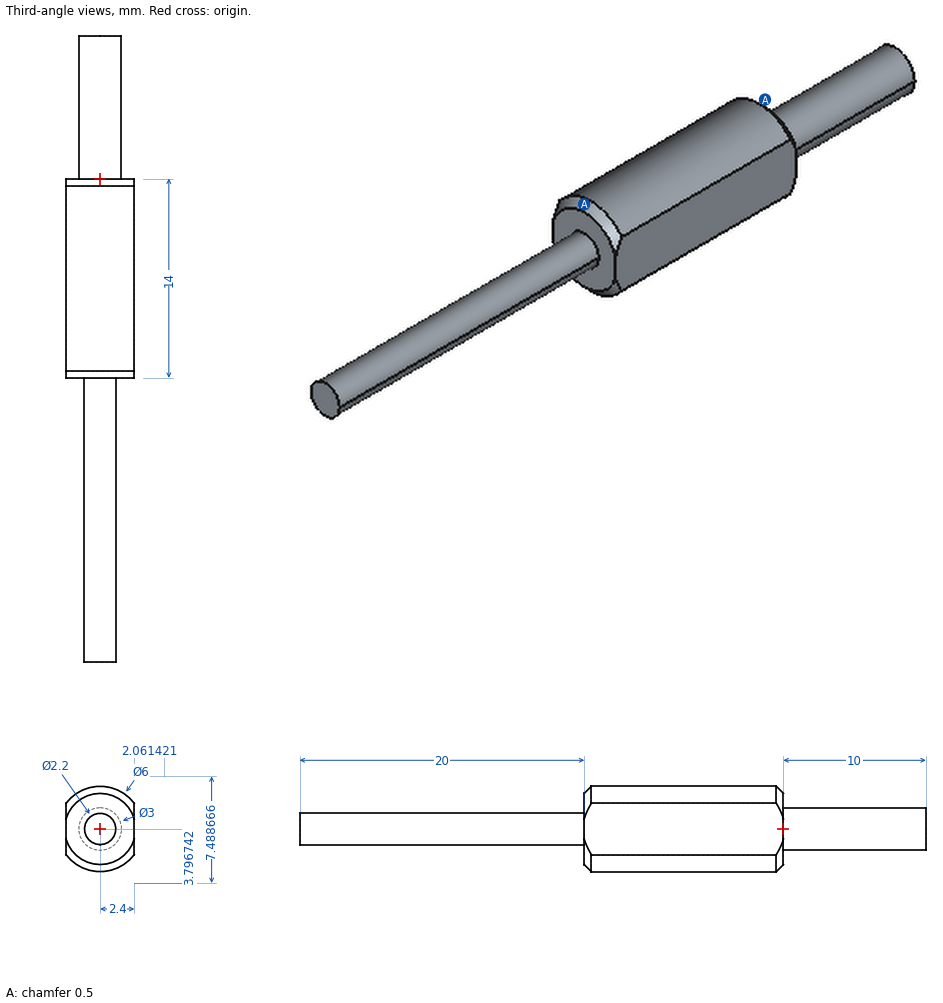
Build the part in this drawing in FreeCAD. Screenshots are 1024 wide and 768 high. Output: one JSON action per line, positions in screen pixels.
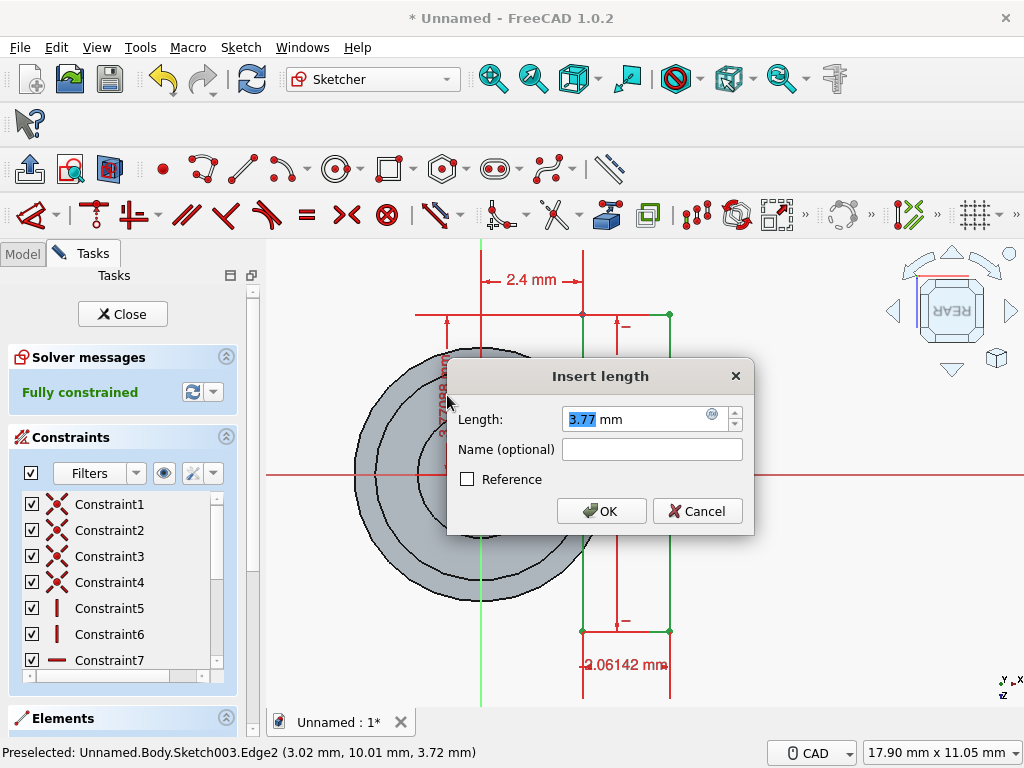
{"action": "type", "text": "3.796742"}
{"action": "key", "text": "Return"}
{"action": "key", "text": "Escape"}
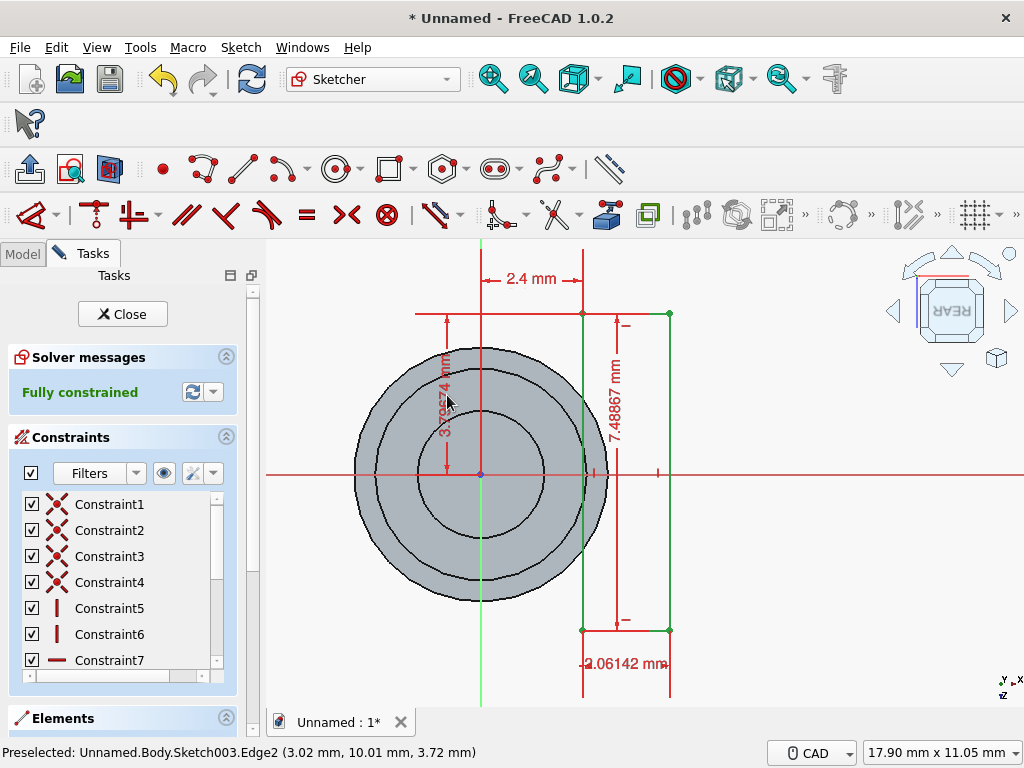
{"action": "left_click", "coordinate": [123, 314]}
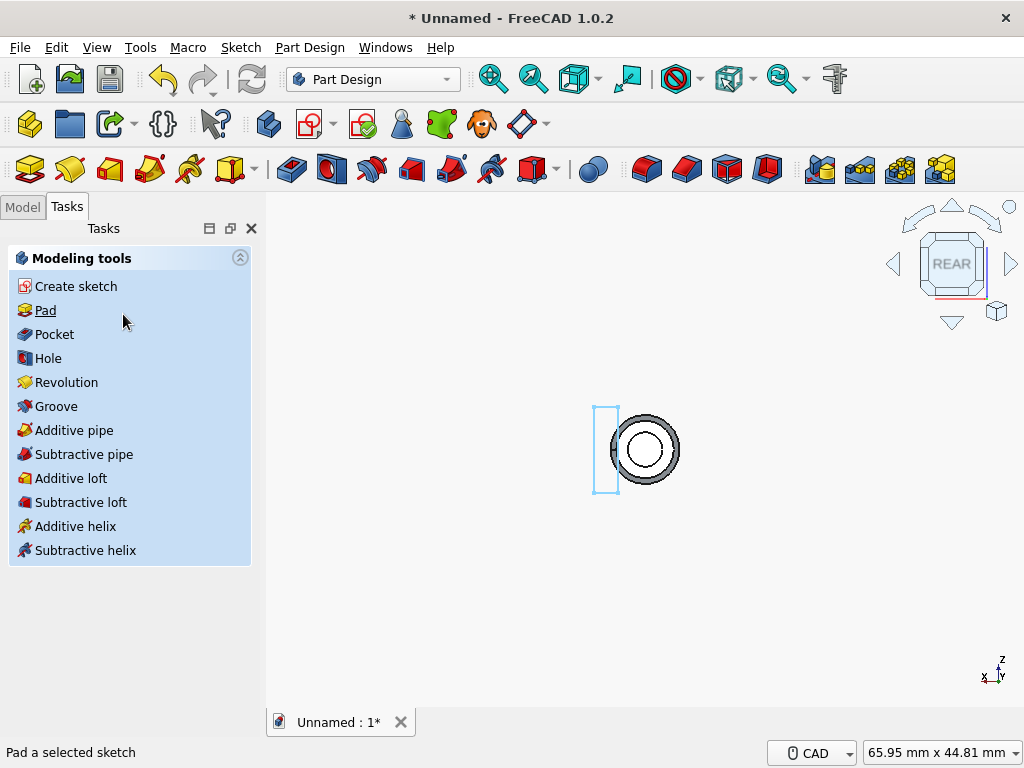
{"action": "left_click", "coordinate": [292, 170]}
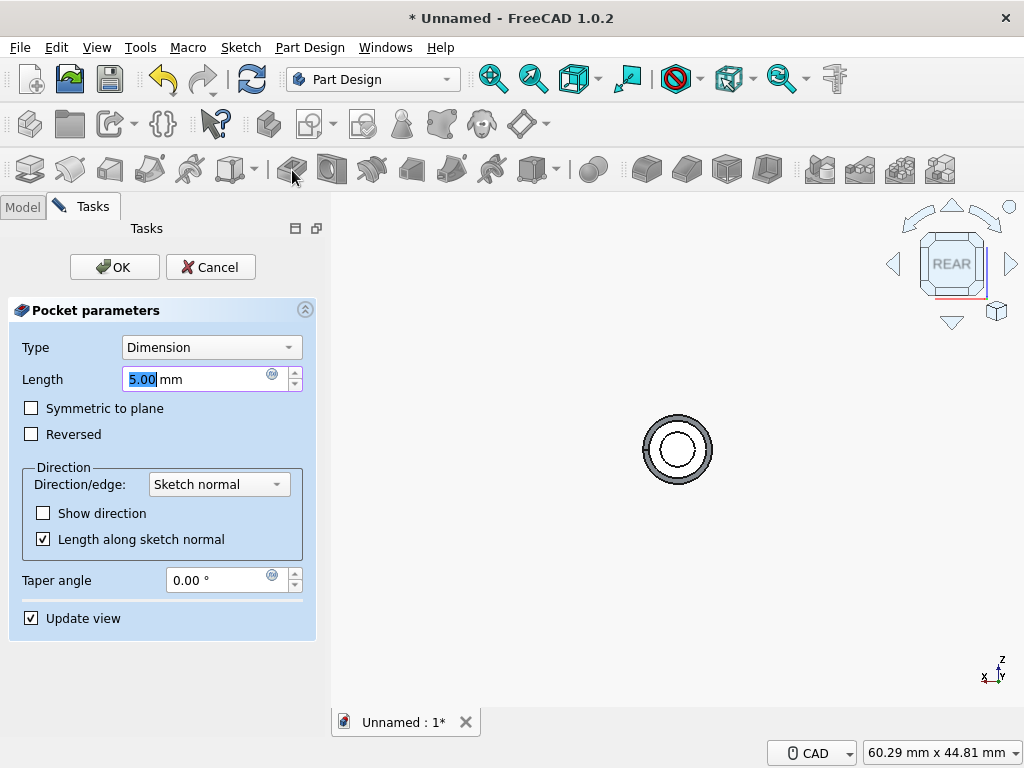
{"action": "left_click", "coordinate": [212, 348]}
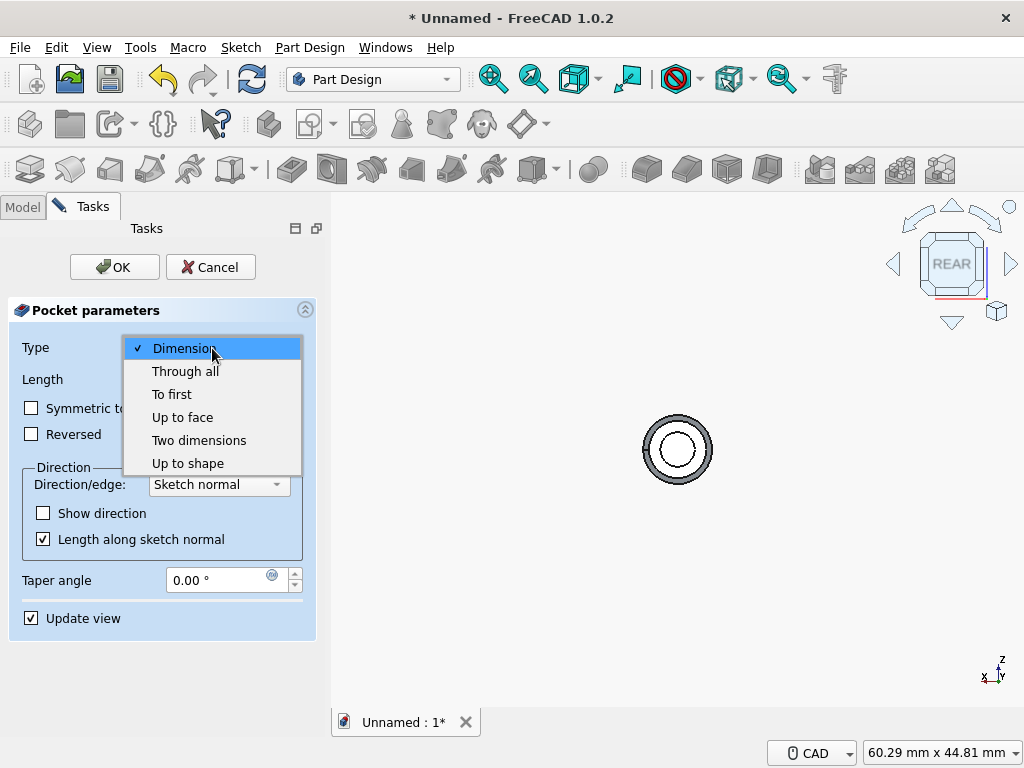
{"action": "left_click", "coordinate": [212, 372]}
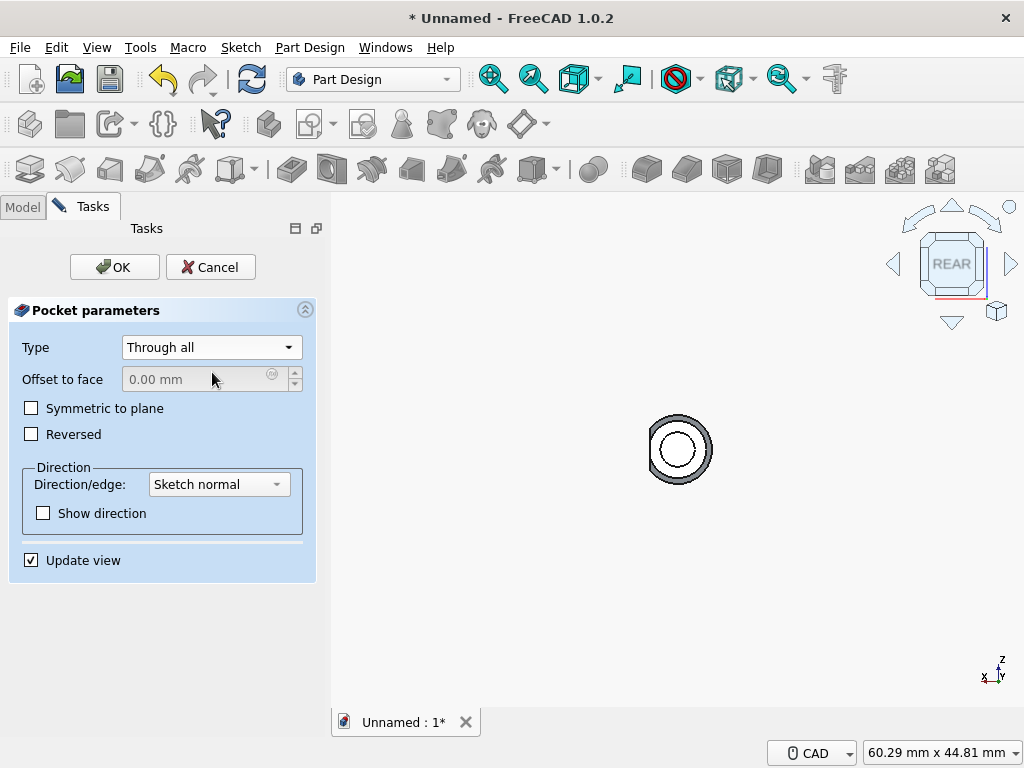
{"action": "left_click", "coordinate": [115, 267]}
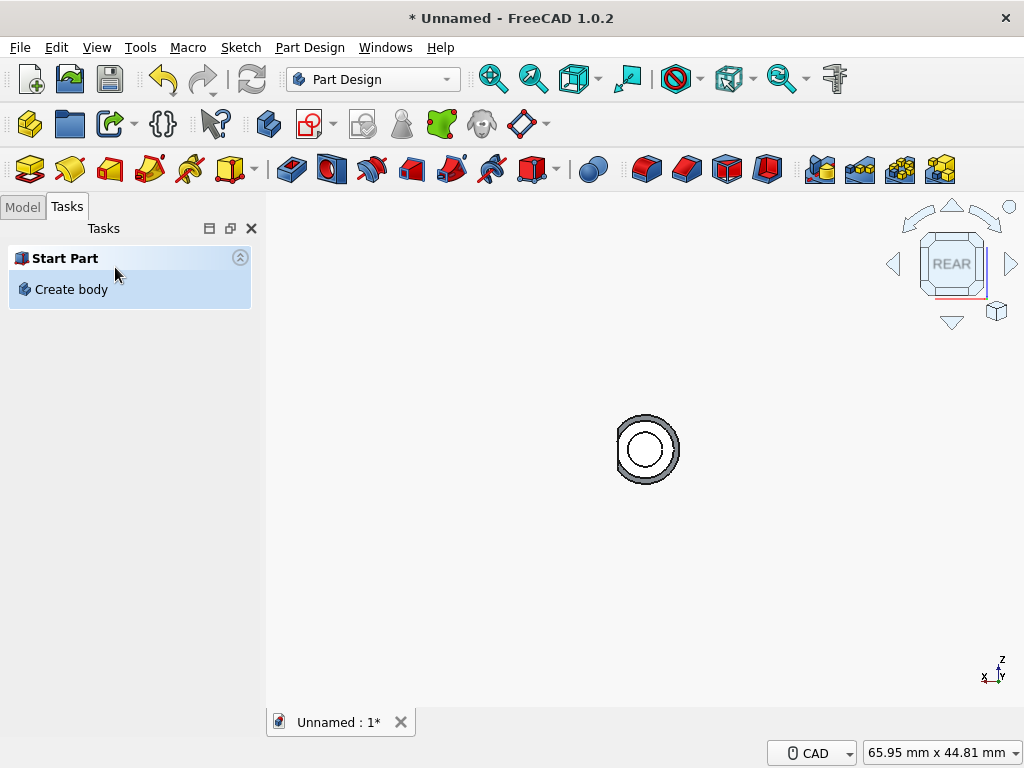
{"action": "left_click", "coordinate": [494, 80]}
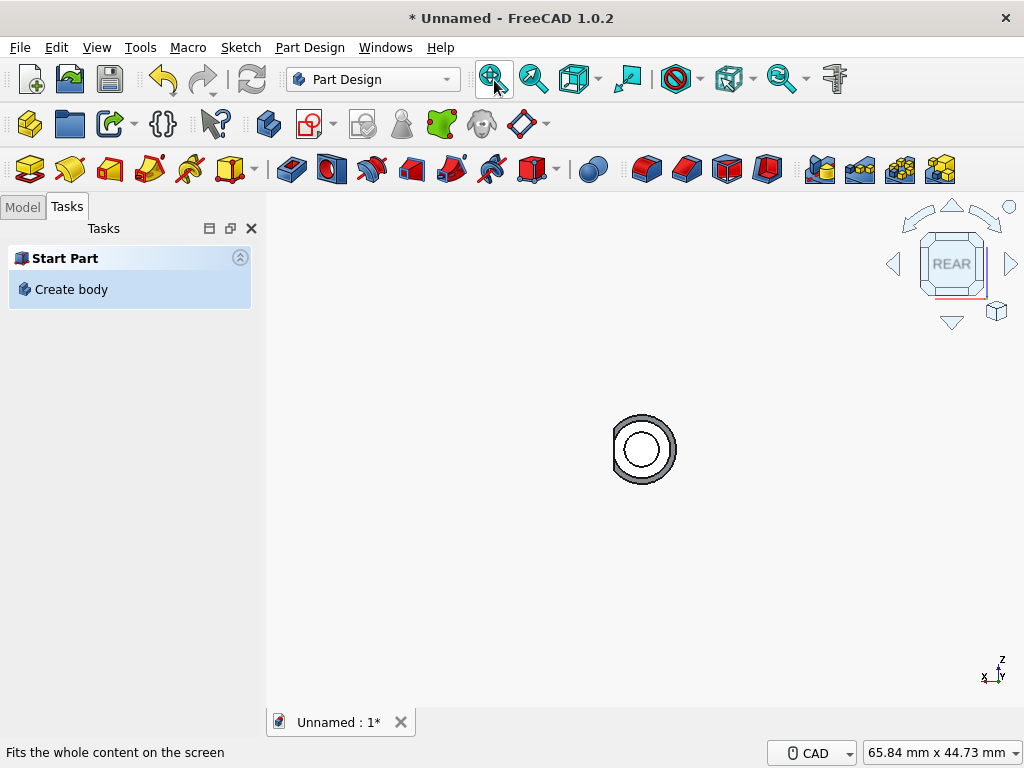
{"action": "left_click", "coordinate": [23, 206]}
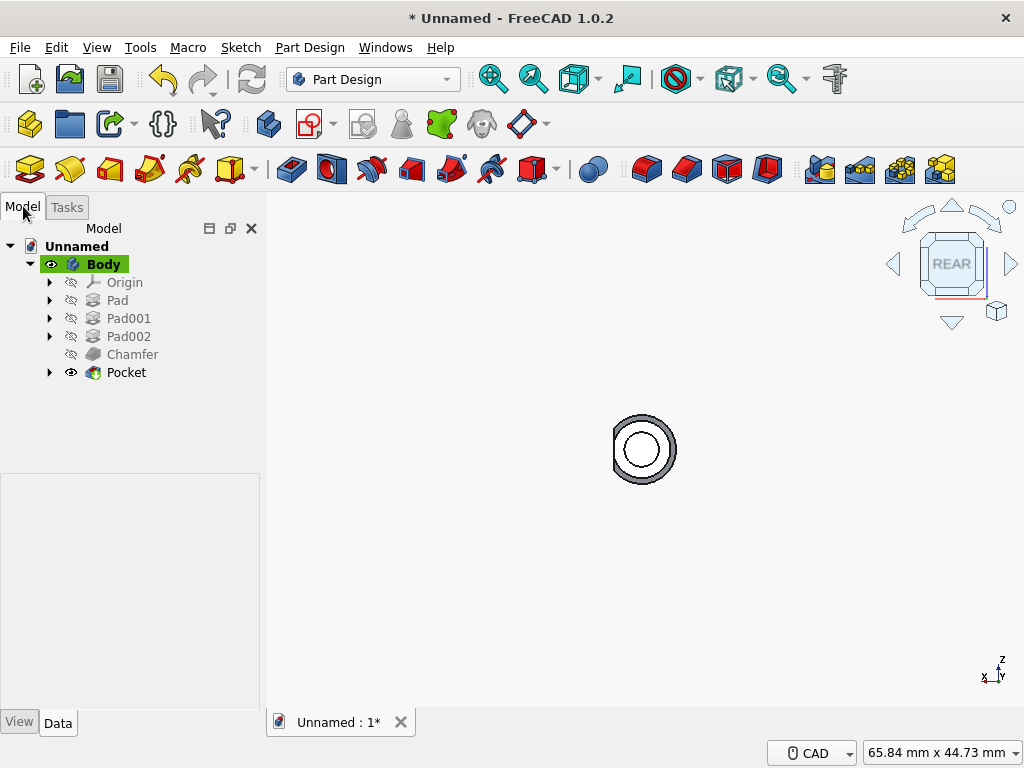
{"action": "left_click", "coordinate": [116, 372]}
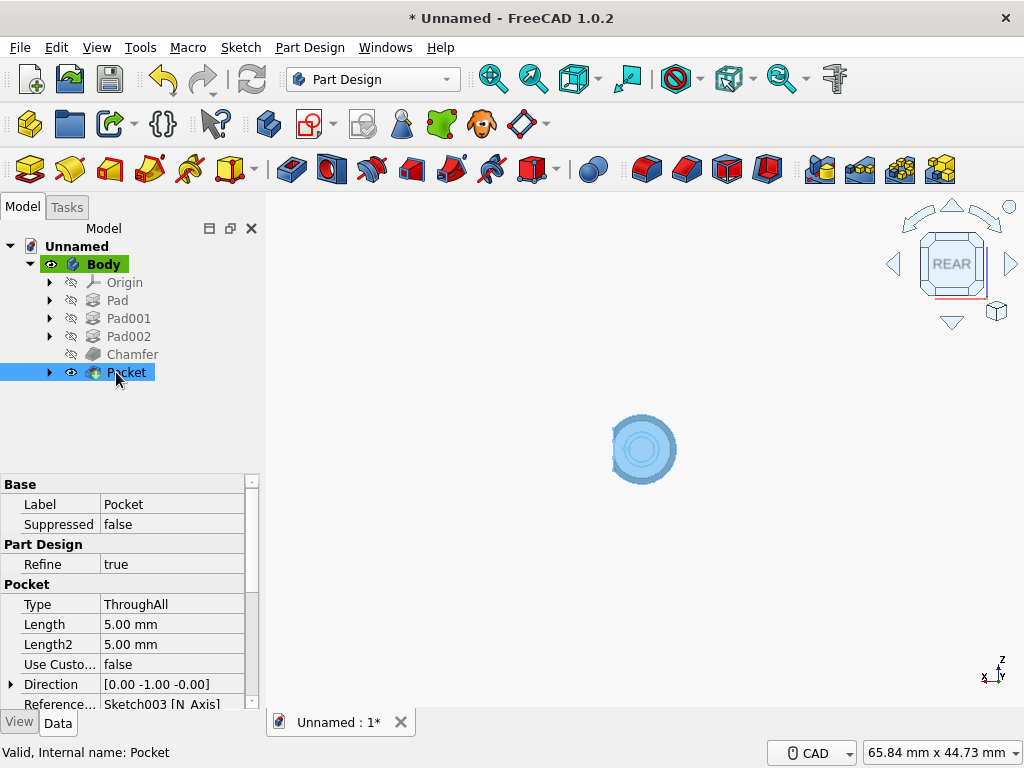
{"action": "left_click", "coordinate": [820, 170]}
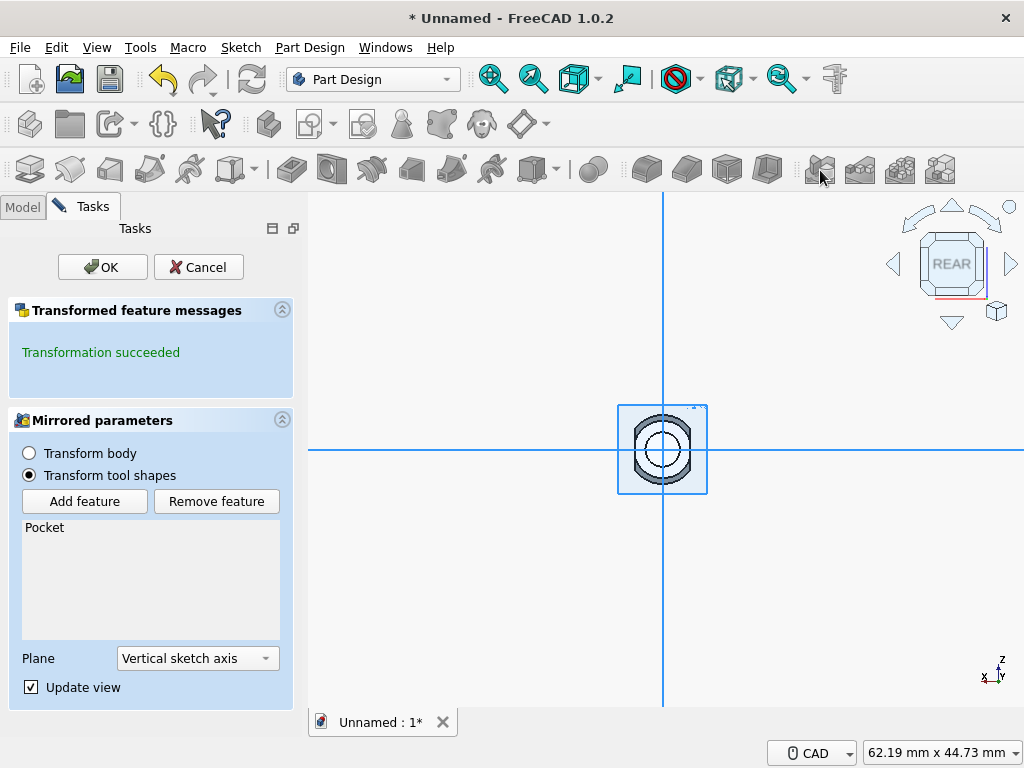
{"action": "left_click", "coordinate": [198, 658]}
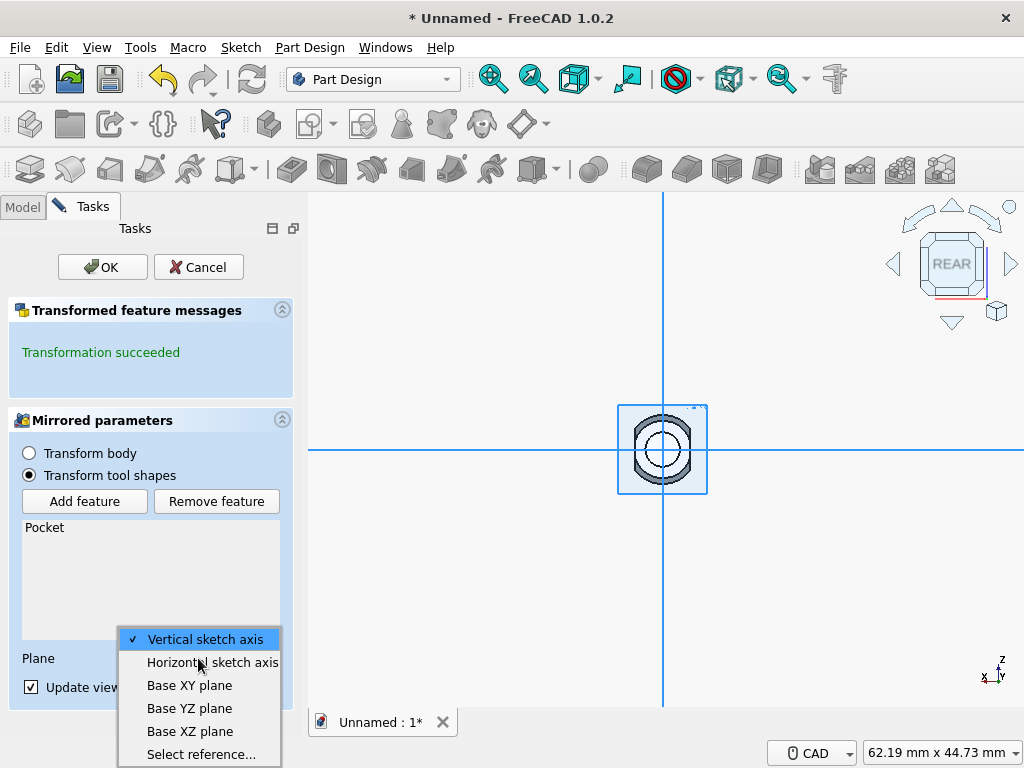
{"action": "left_click", "coordinate": [198, 708]}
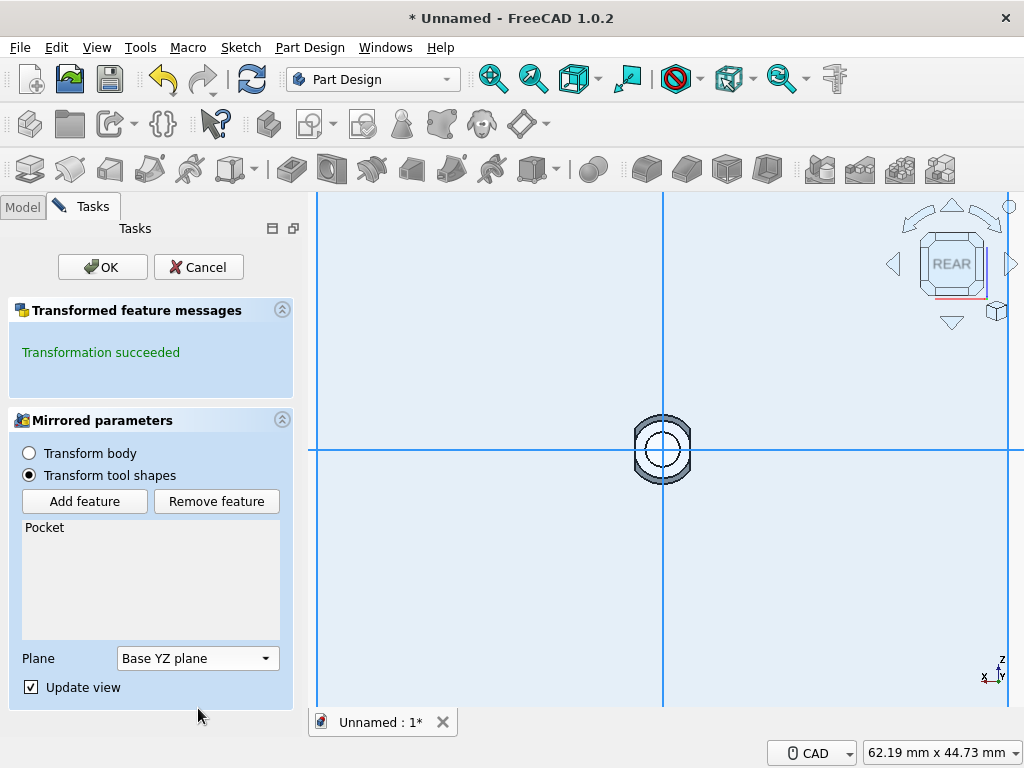
{"action": "left_click", "coordinate": [103, 267]}